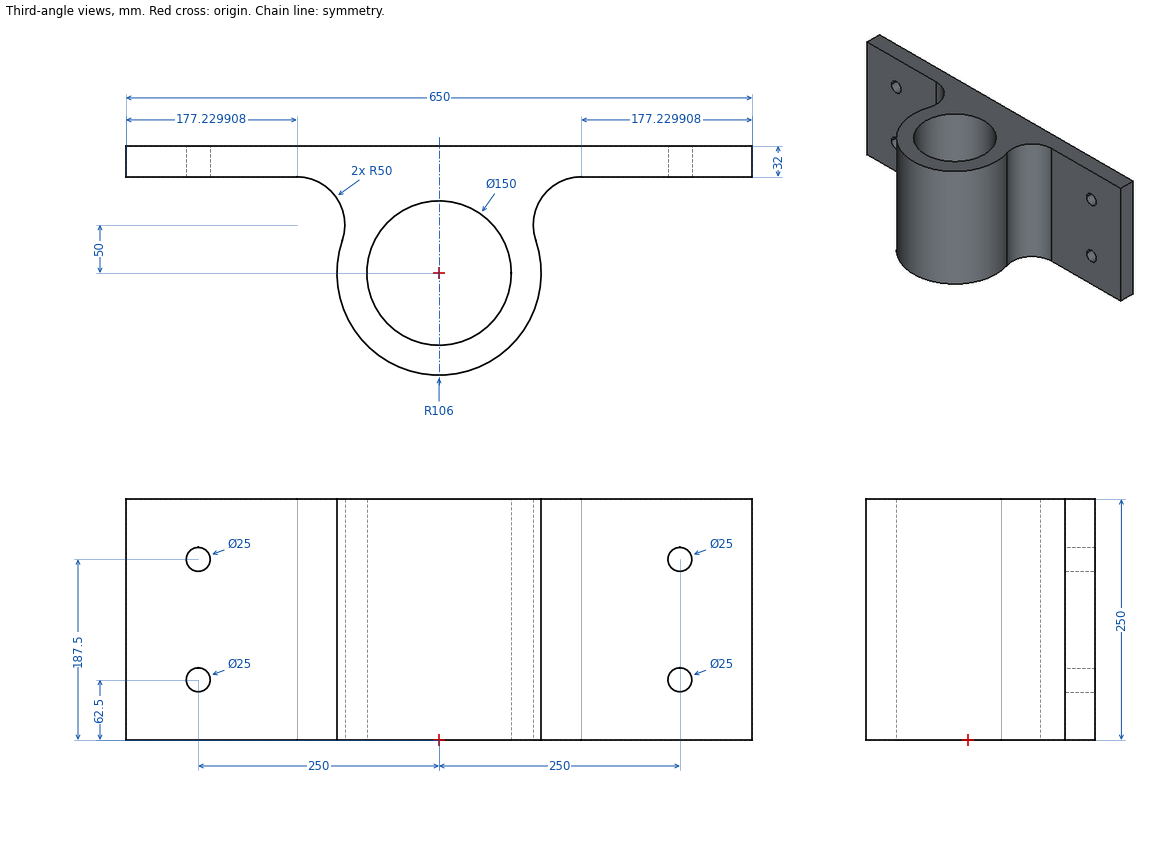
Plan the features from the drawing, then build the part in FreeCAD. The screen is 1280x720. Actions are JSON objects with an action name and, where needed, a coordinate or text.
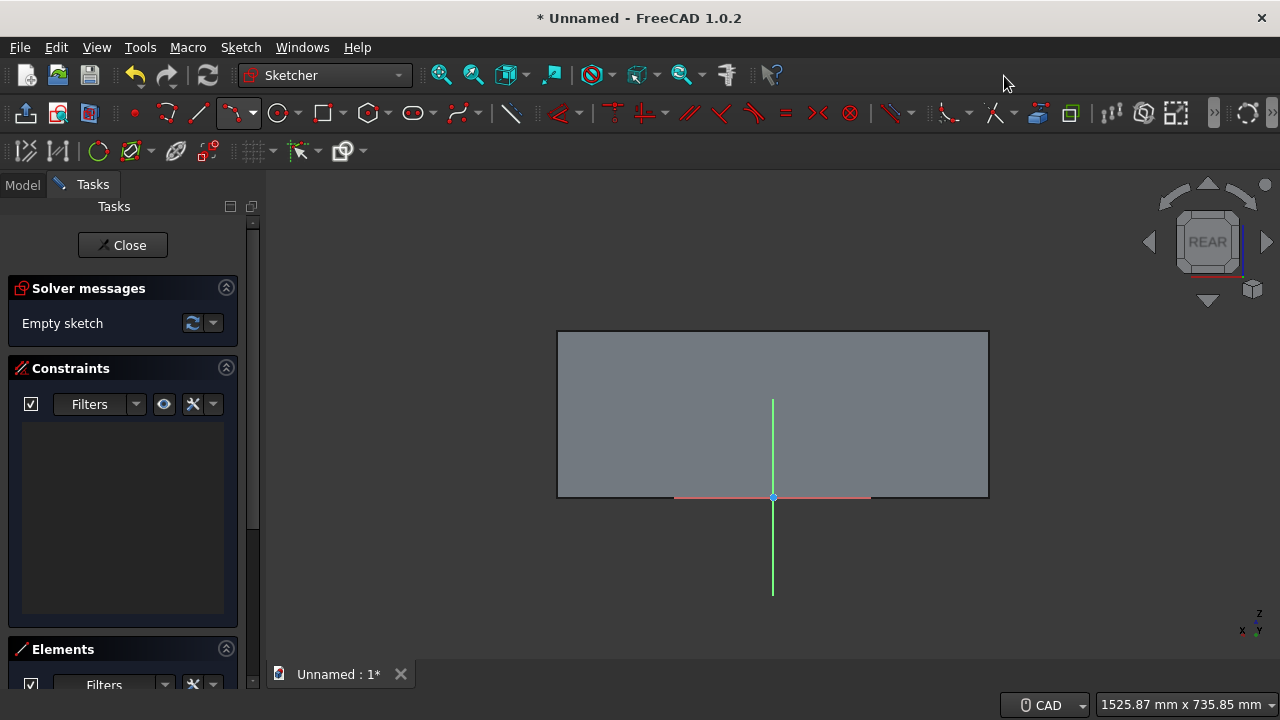
{"action": "scroll", "coordinate": [951, 458], "scroll_direction": "up", "scroll_amount": 15}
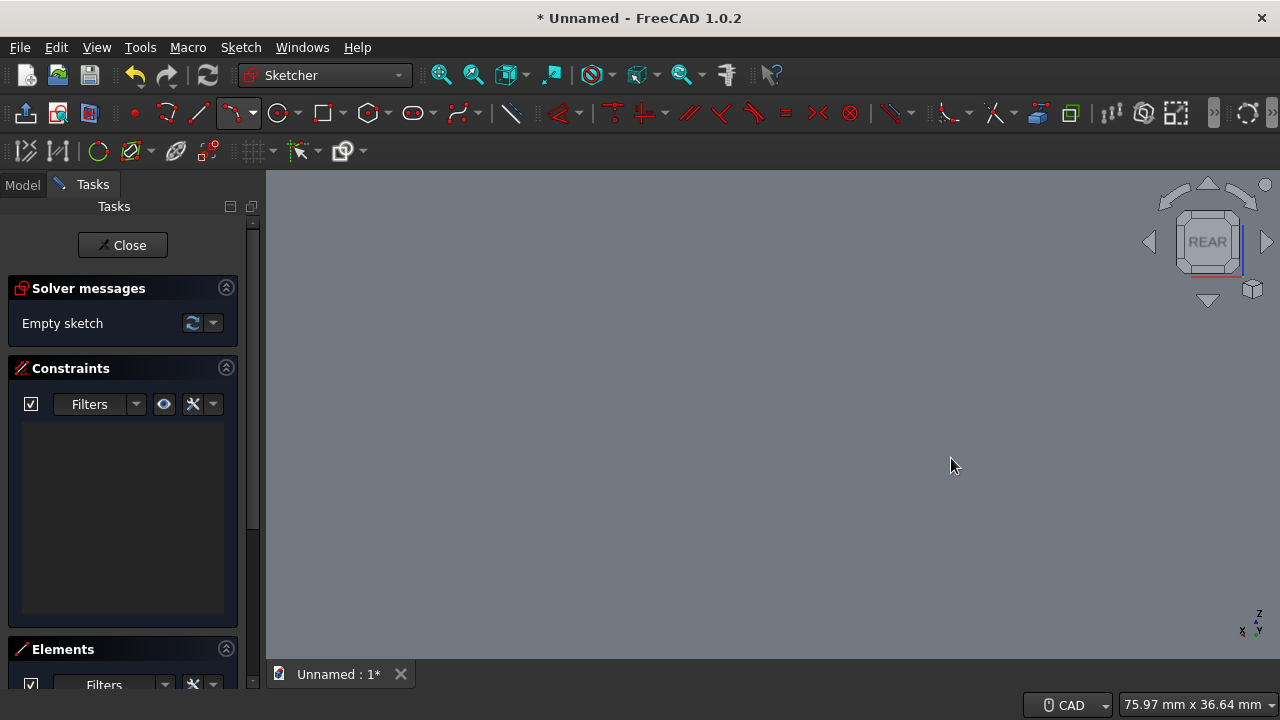
{"action": "key", "text": "g c"}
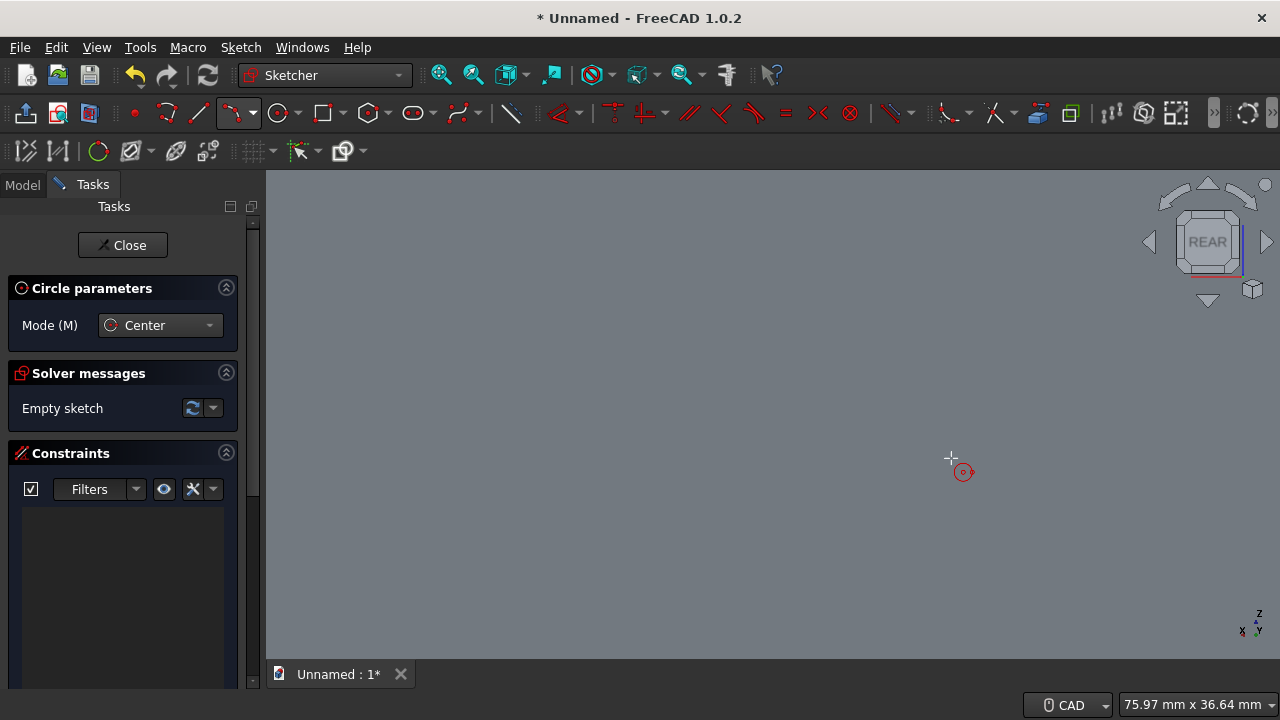
{"action": "left_click", "coordinate": [700, 407]}
{"action": "mouse_move", "coordinate": [818, 289]}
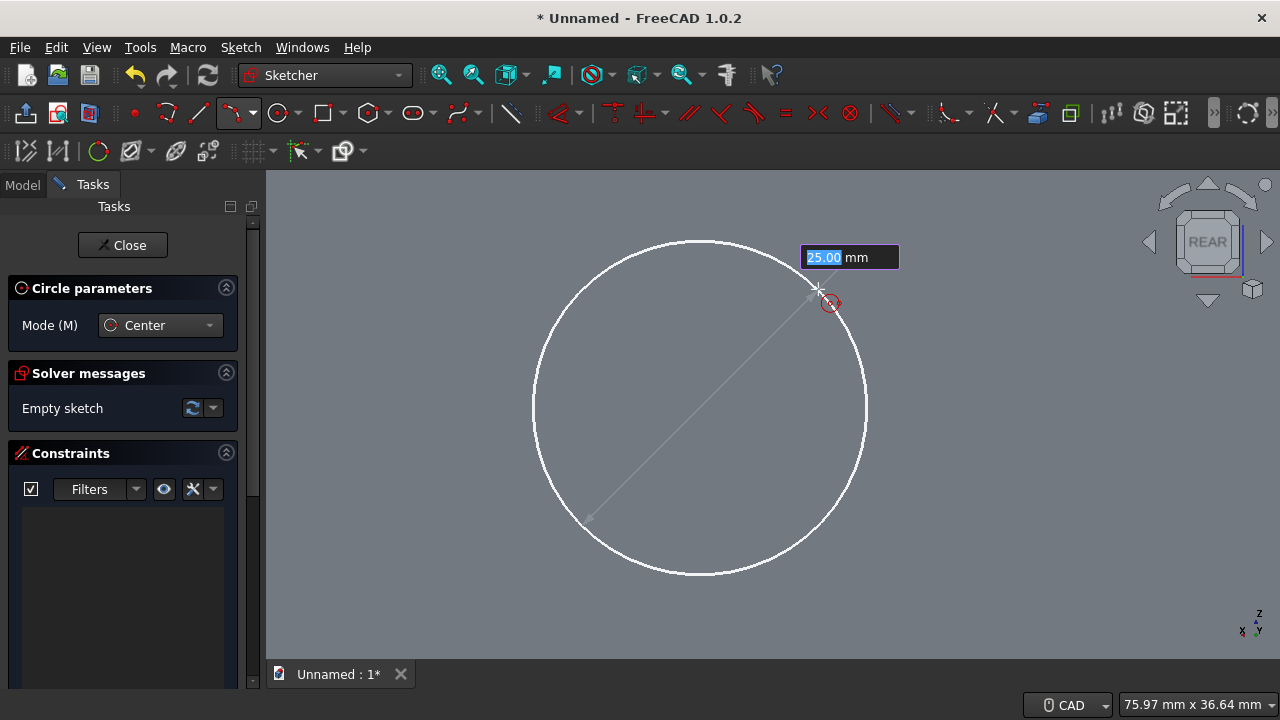
{"action": "type", "text": "25"}
{"action": "key", "text": "Return"}
{"action": "key", "text": "Escape"}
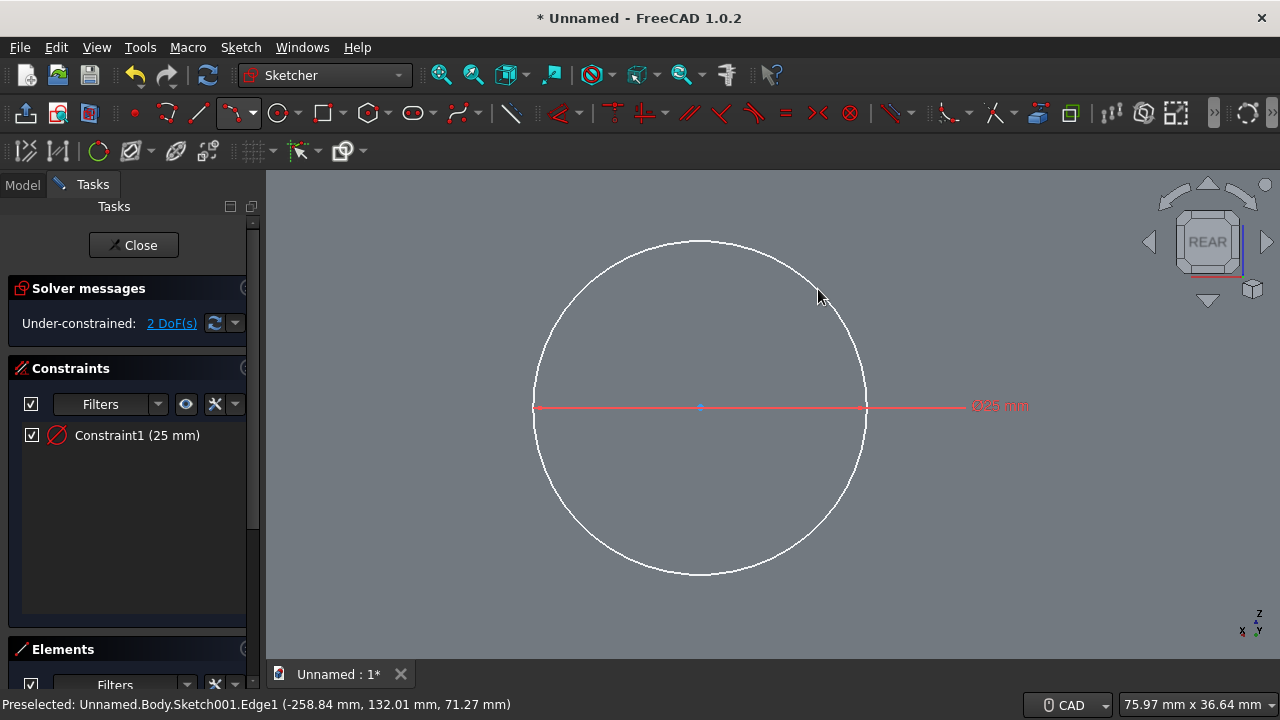
{"action": "left_click", "coordinate": [558, 114]}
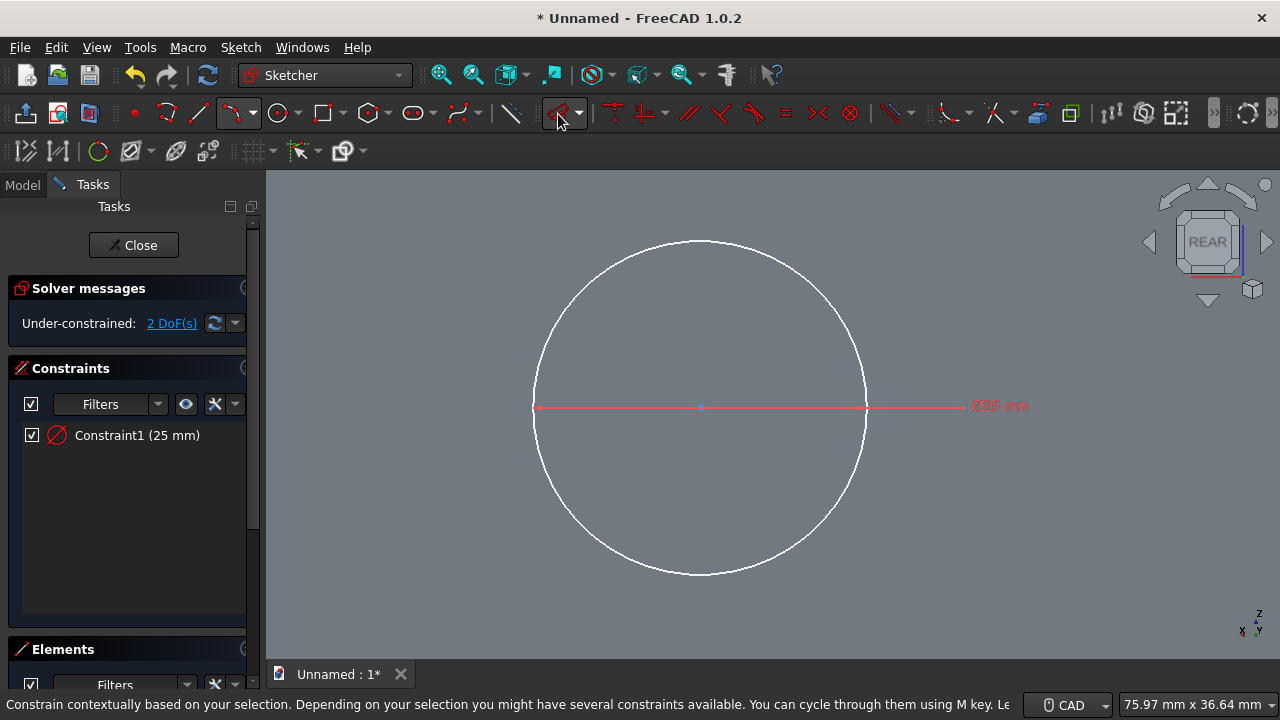
{"action": "left_click", "coordinate": [700, 408]}
{"action": "left_click", "coordinate": [497, 374]}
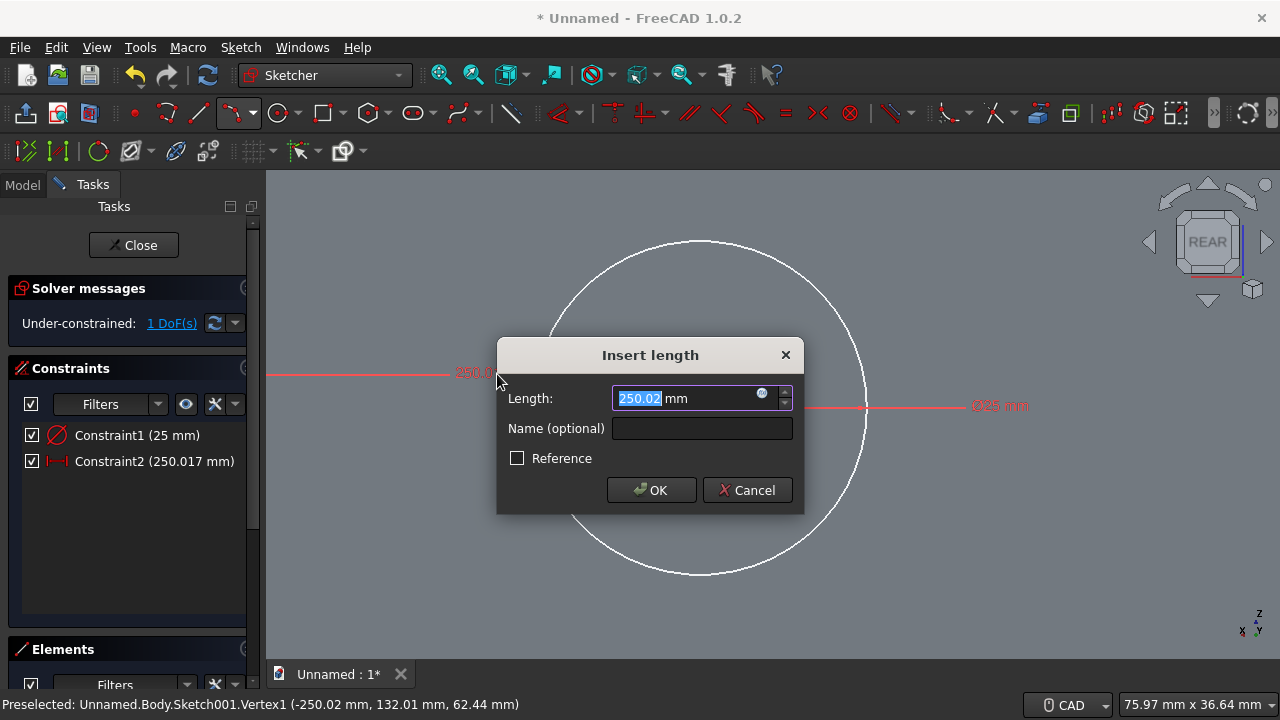
{"action": "type", "text": "250"}
{"action": "key", "text": "Return"}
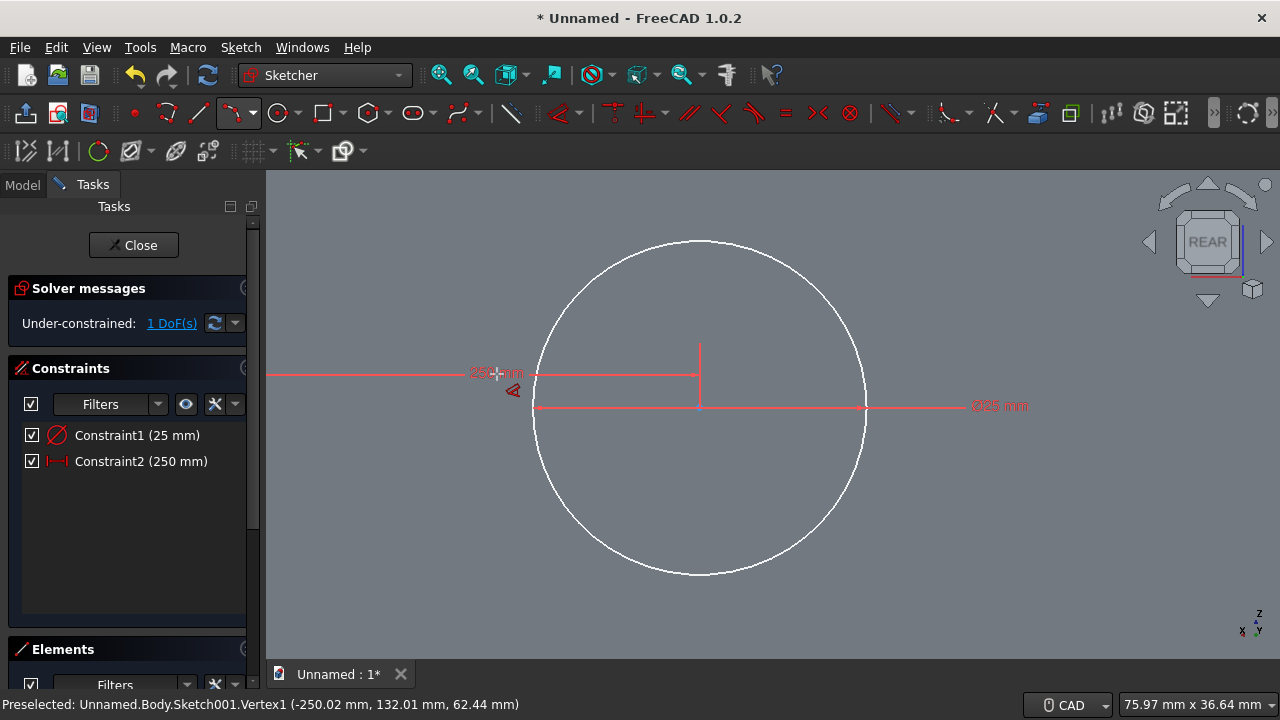
{"action": "left_click", "coordinate": [700, 408]}
{"action": "left_click", "coordinate": [734, 520]}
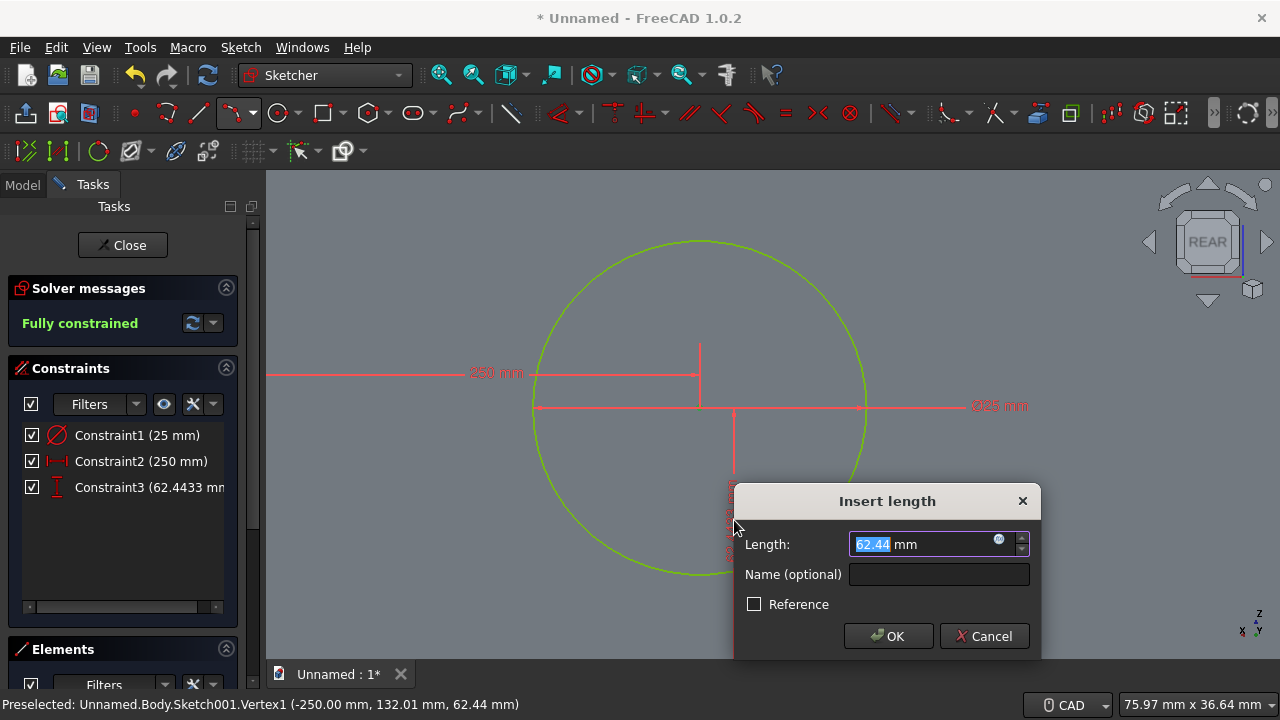
{"action": "type", "text": "62.5"}
{"action": "key", "text": "Return"}
{"action": "key", "text": "Escape"}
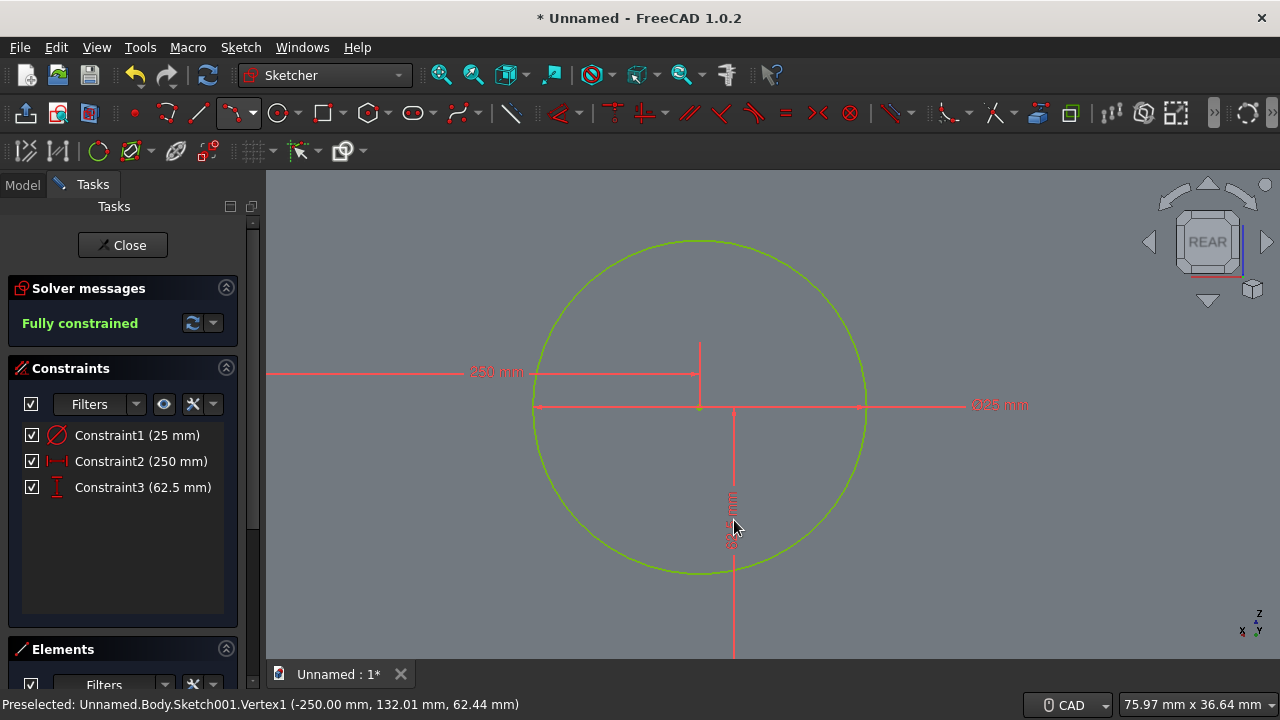
{"action": "left_click", "coordinate": [123, 245]}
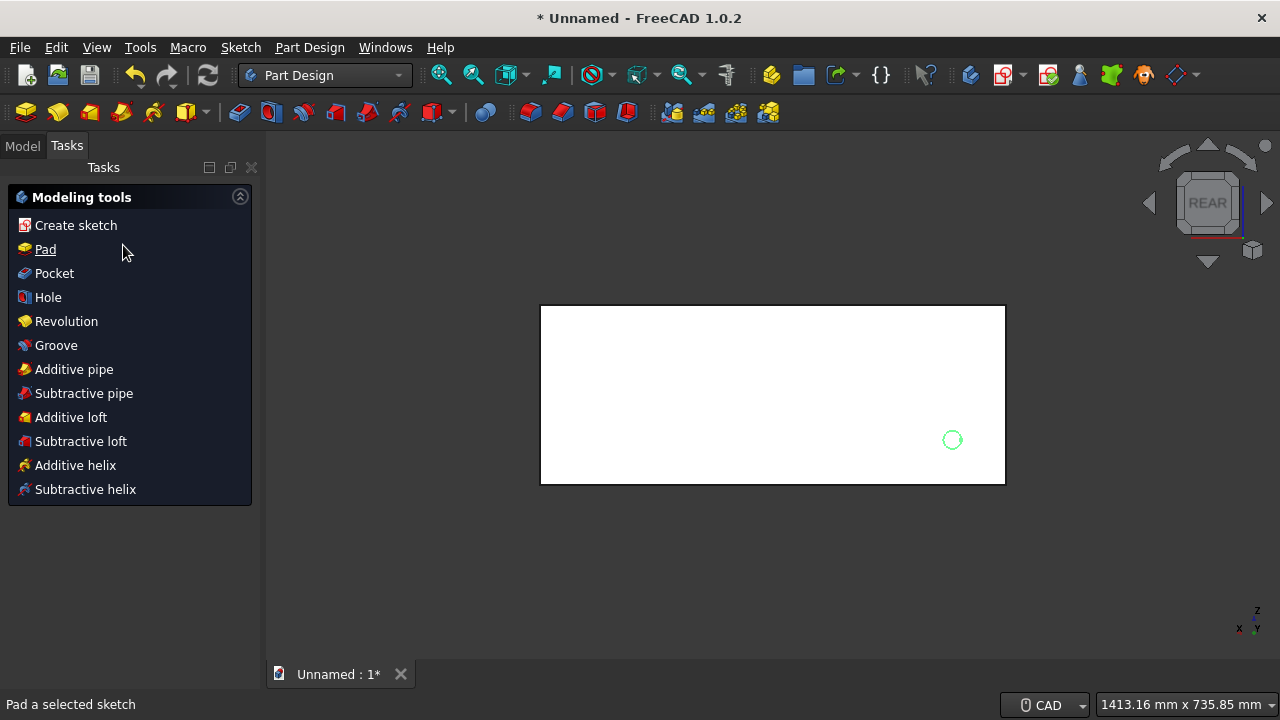
{"action": "left_click", "coordinate": [240, 112]}